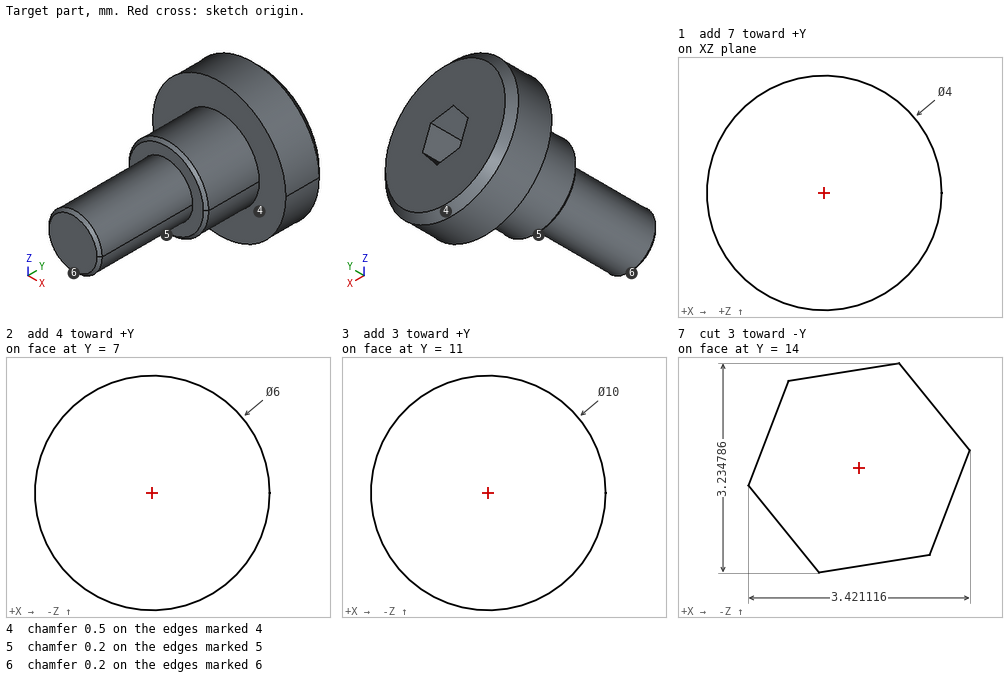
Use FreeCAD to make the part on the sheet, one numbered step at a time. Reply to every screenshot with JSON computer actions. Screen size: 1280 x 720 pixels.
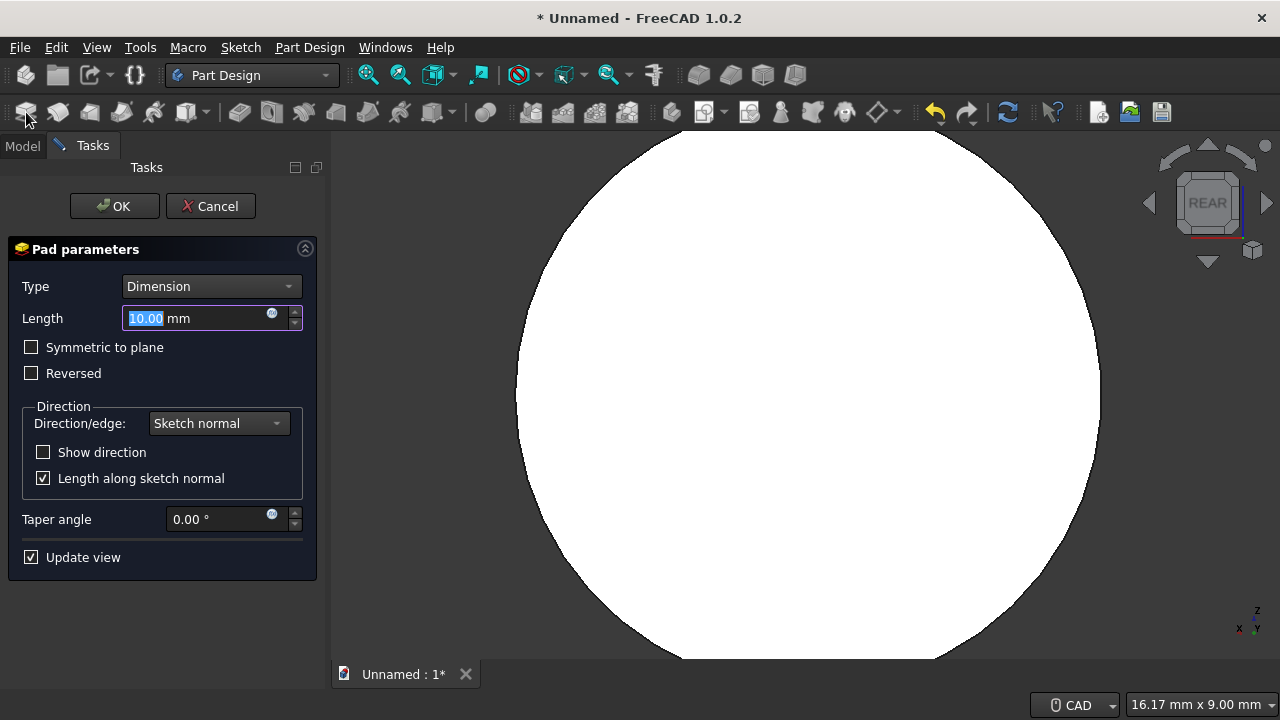
{"action": "type", "text": "3"}
{"action": "key", "text": "Tab"}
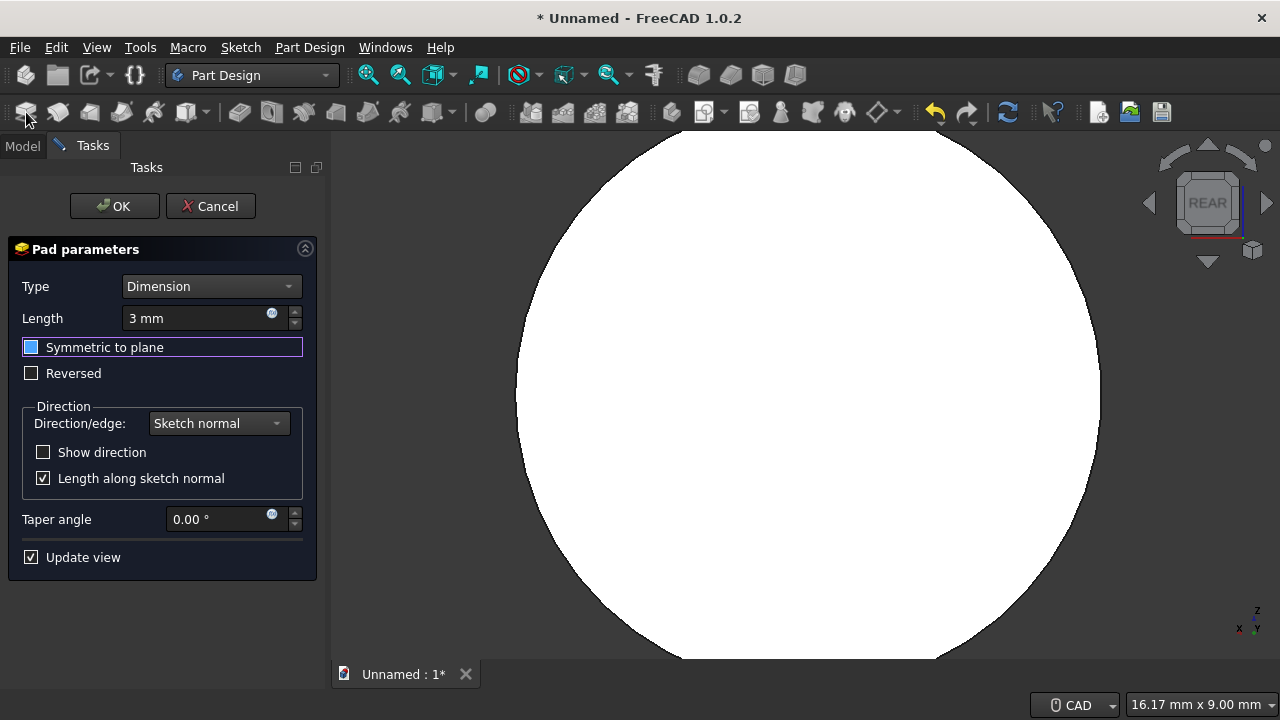
{"action": "left_click", "coordinate": [115, 206]}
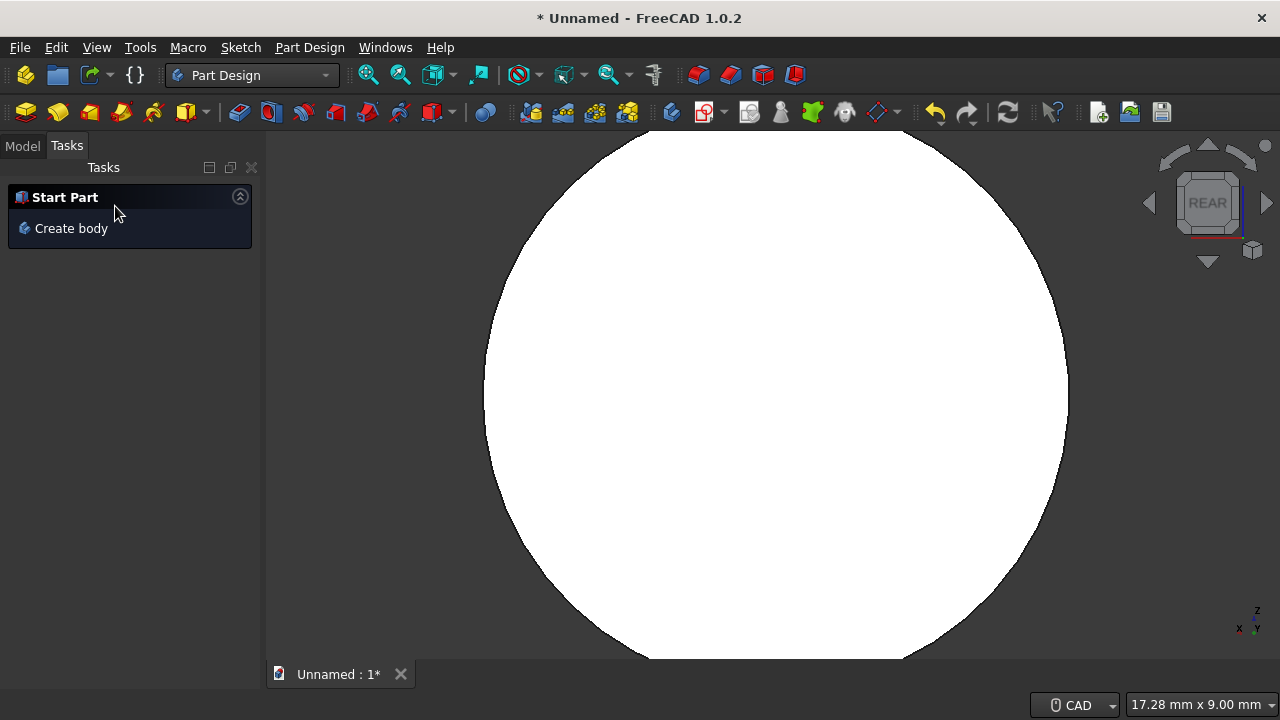
{"action": "key", "text": "v f"}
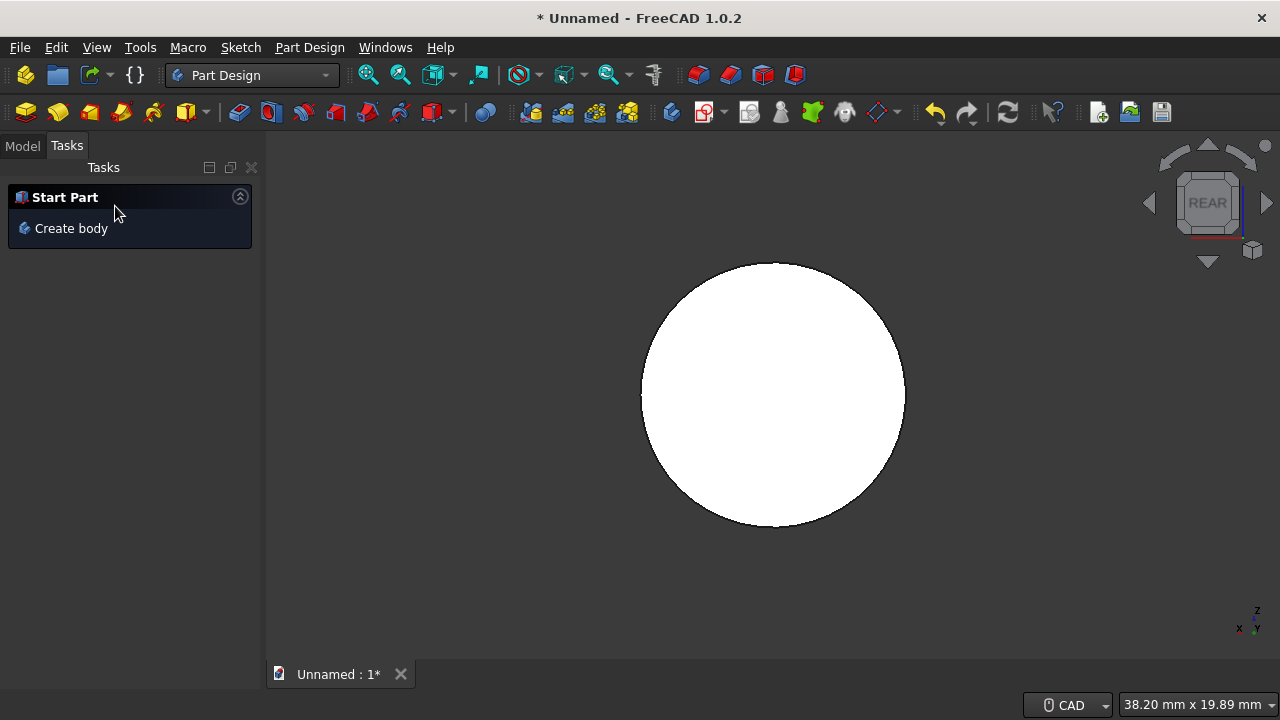
{"action": "left_click", "coordinate": [906, 394]}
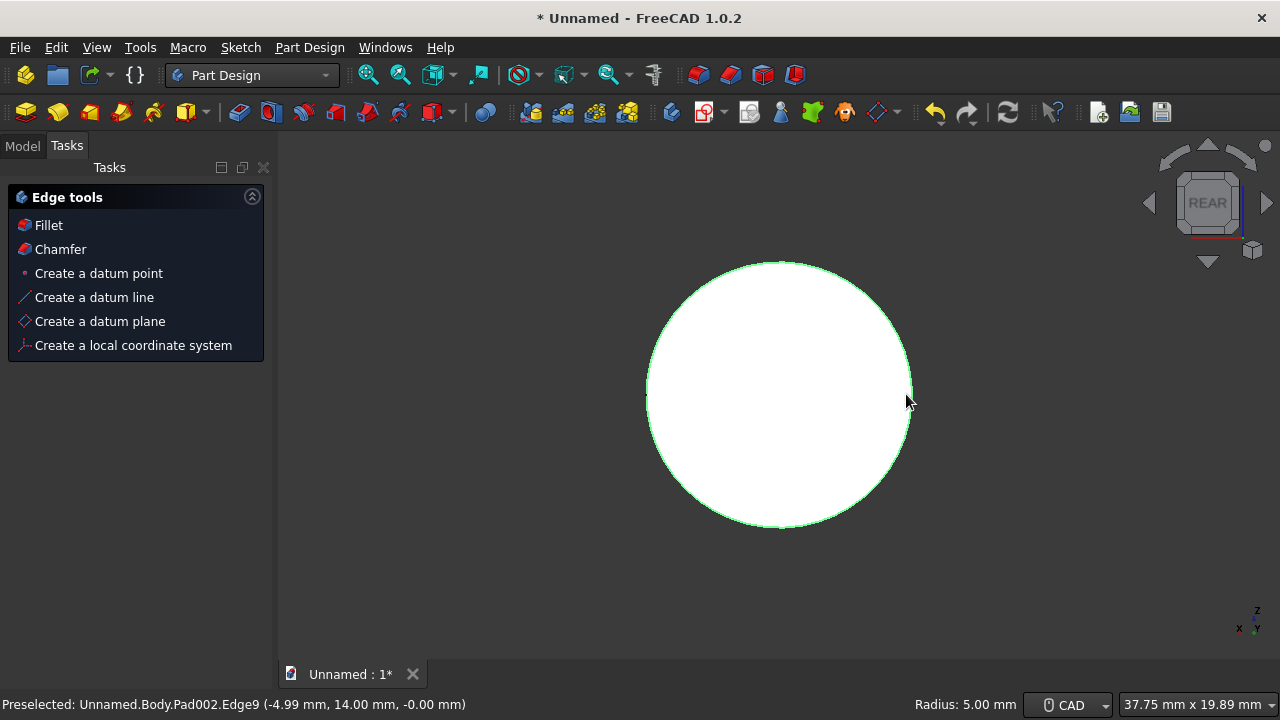
{"action": "left_click", "coordinate": [732, 76]}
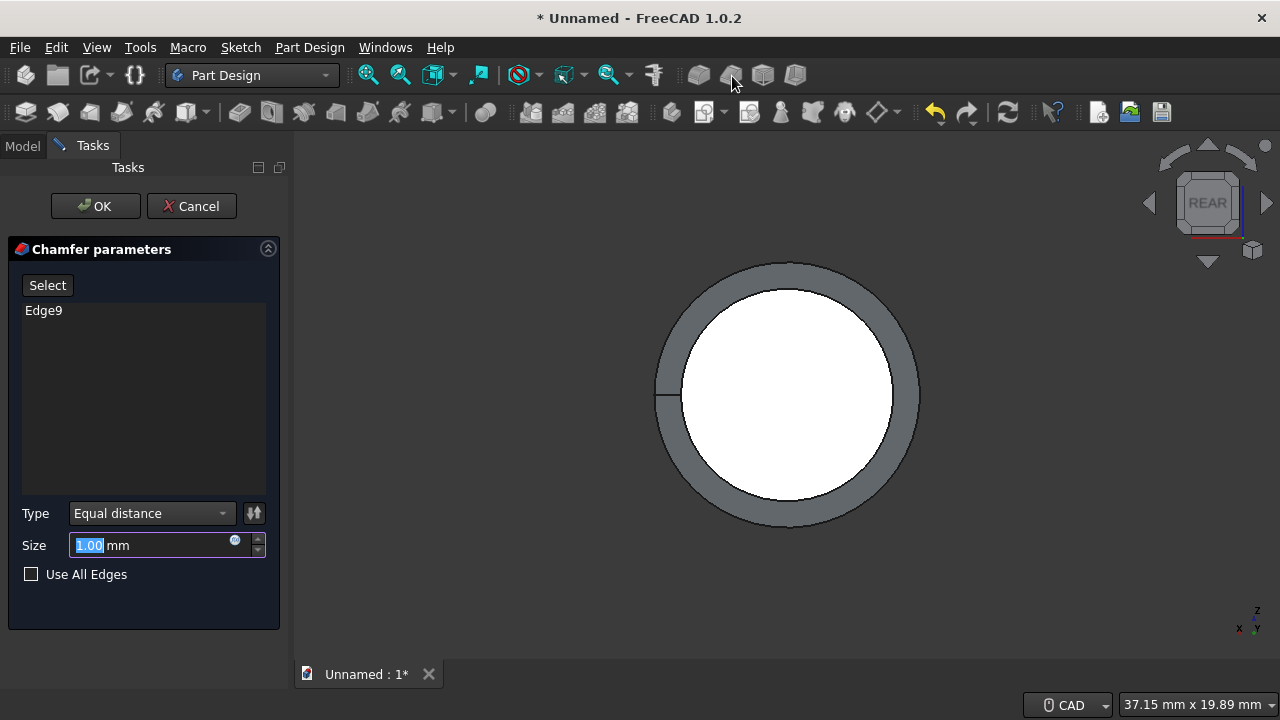
{"action": "type", "text": "0.5"}
{"action": "key", "text": "Tab"}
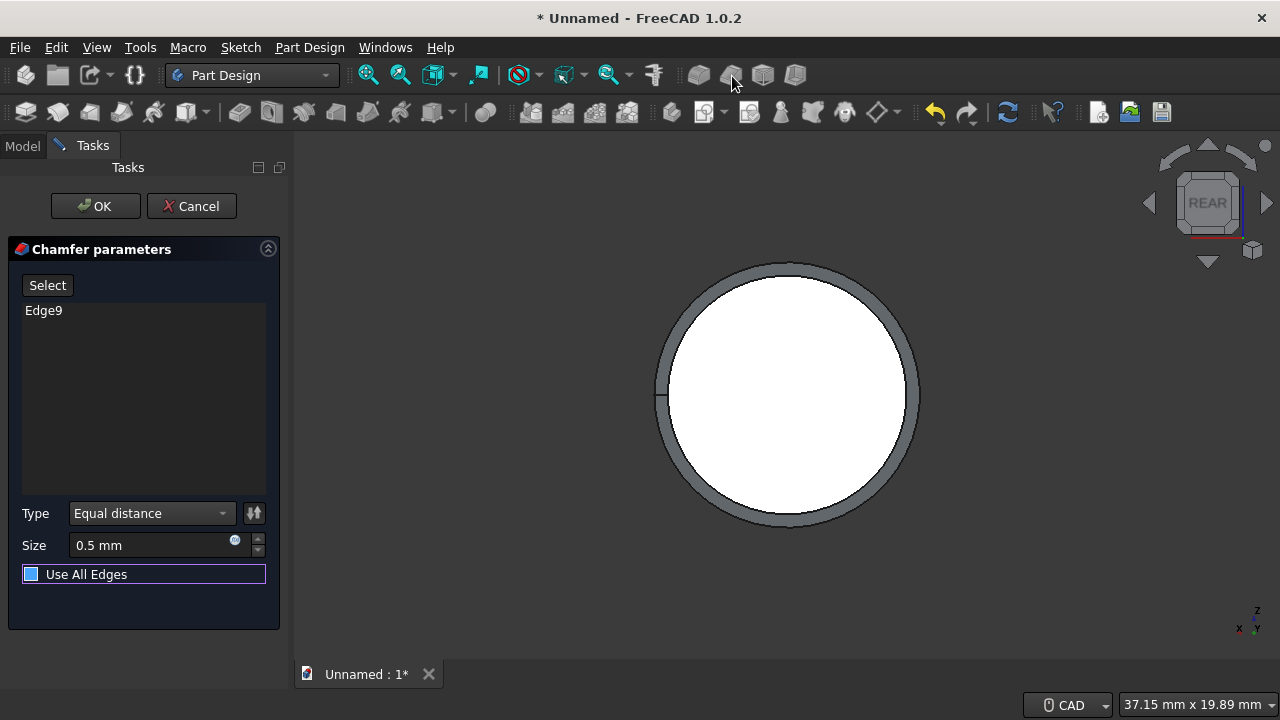
{"action": "left_click", "coordinate": [96, 206]}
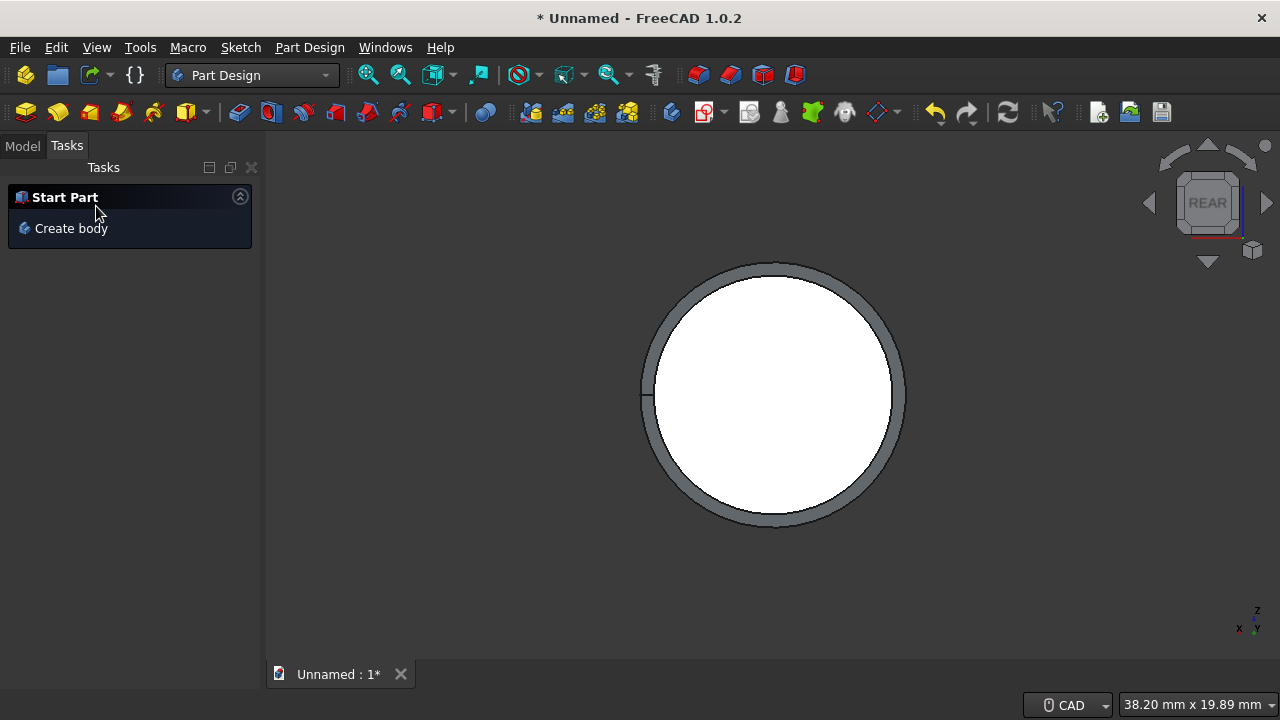
{"action": "key", "text": "0"}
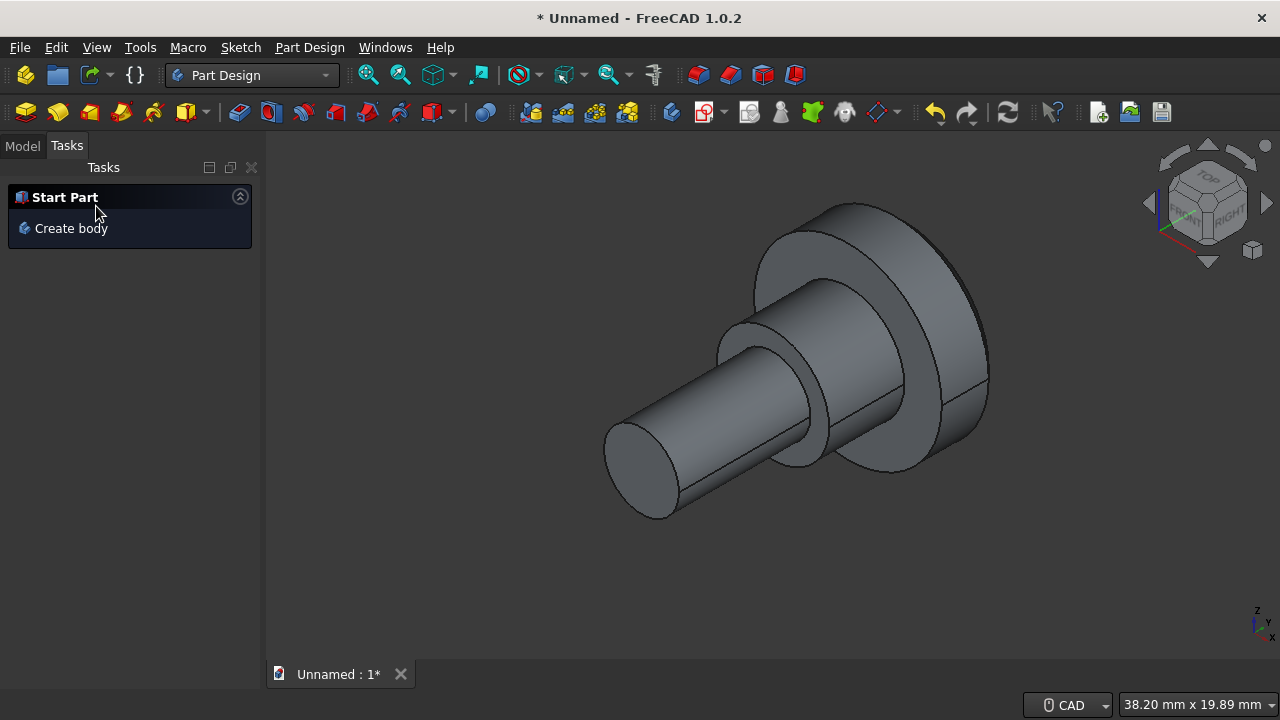
{"action": "left_click", "coordinate": [755, 322]}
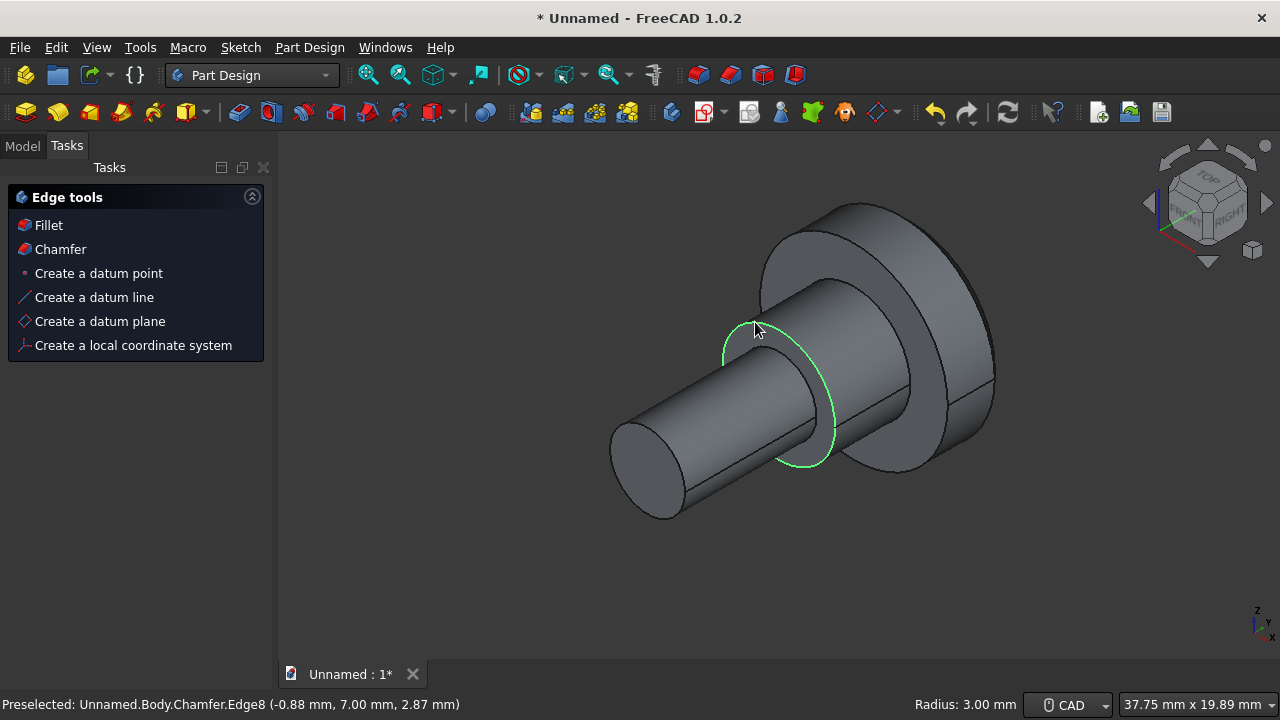
{"action": "left_click", "coordinate": [732, 76]}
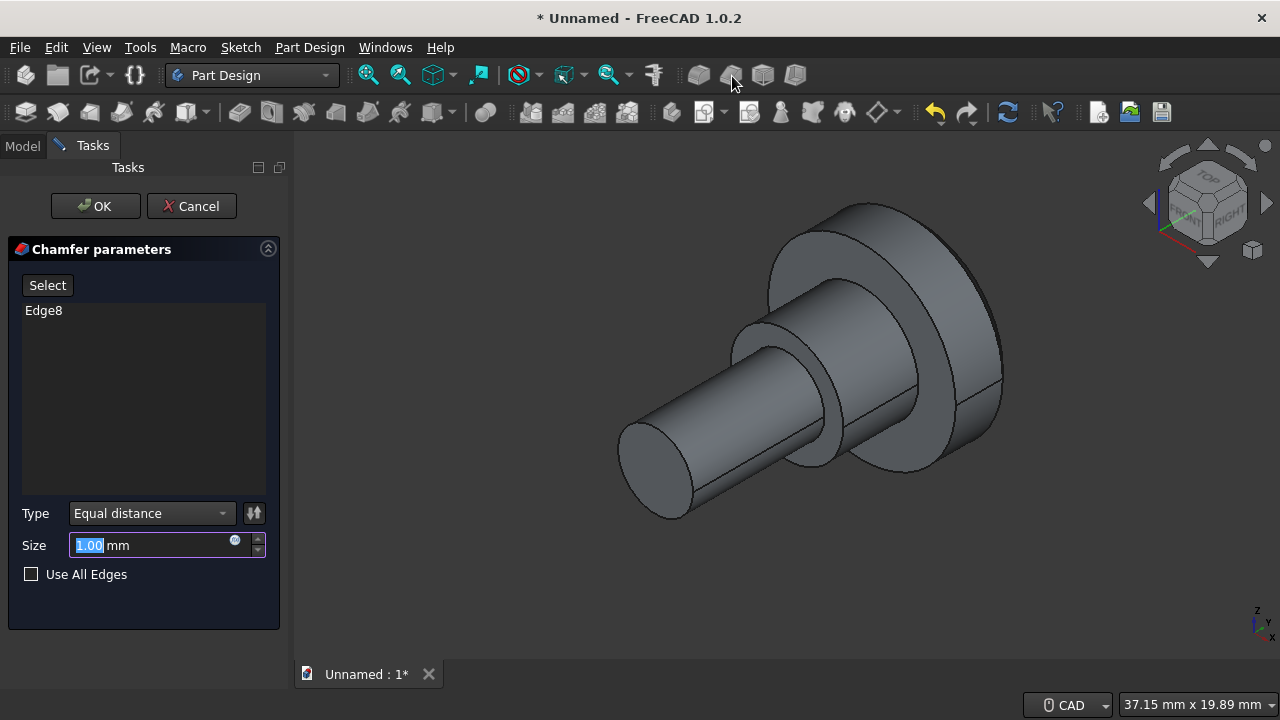
{"action": "type", "text": "0.2"}
{"action": "key", "text": "Tab"}